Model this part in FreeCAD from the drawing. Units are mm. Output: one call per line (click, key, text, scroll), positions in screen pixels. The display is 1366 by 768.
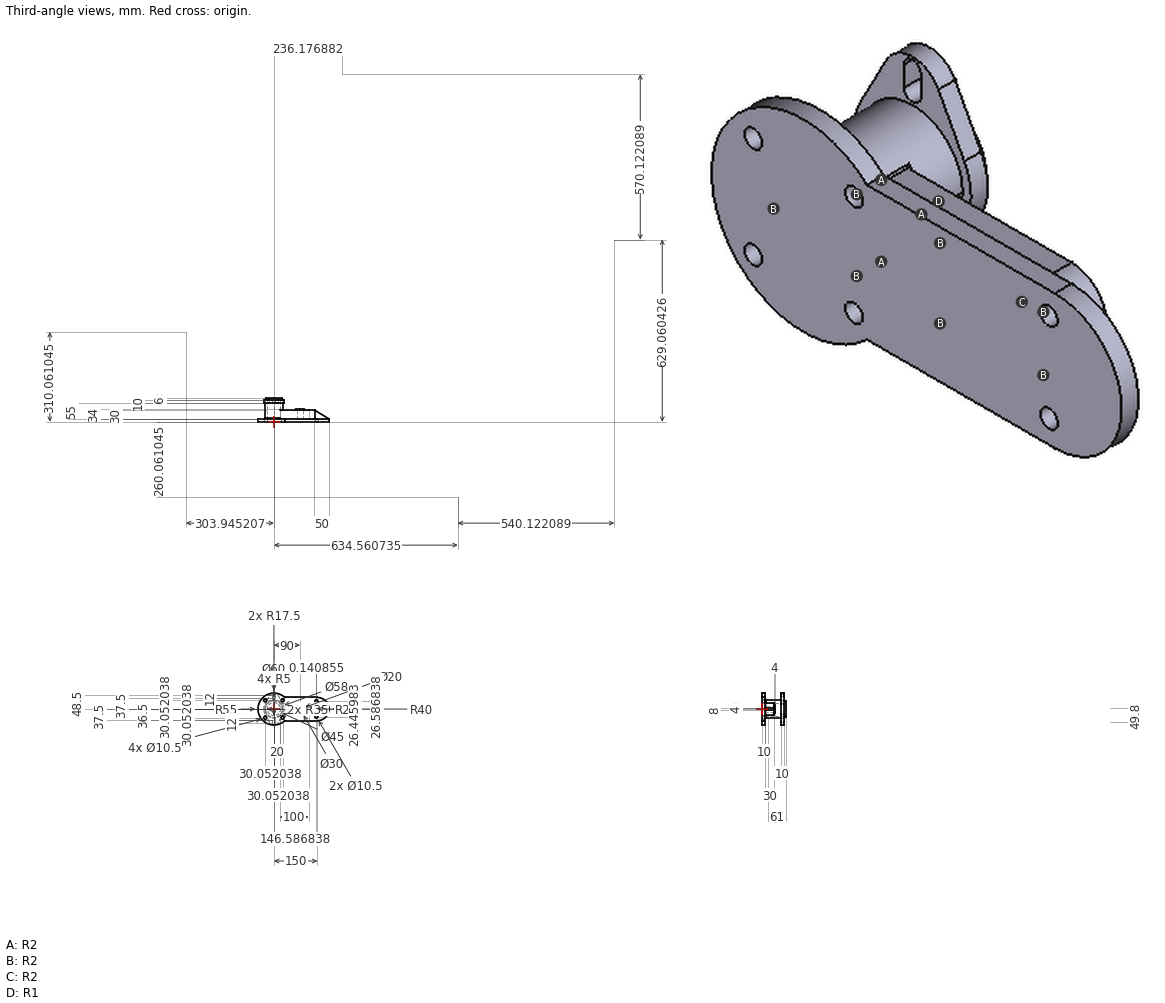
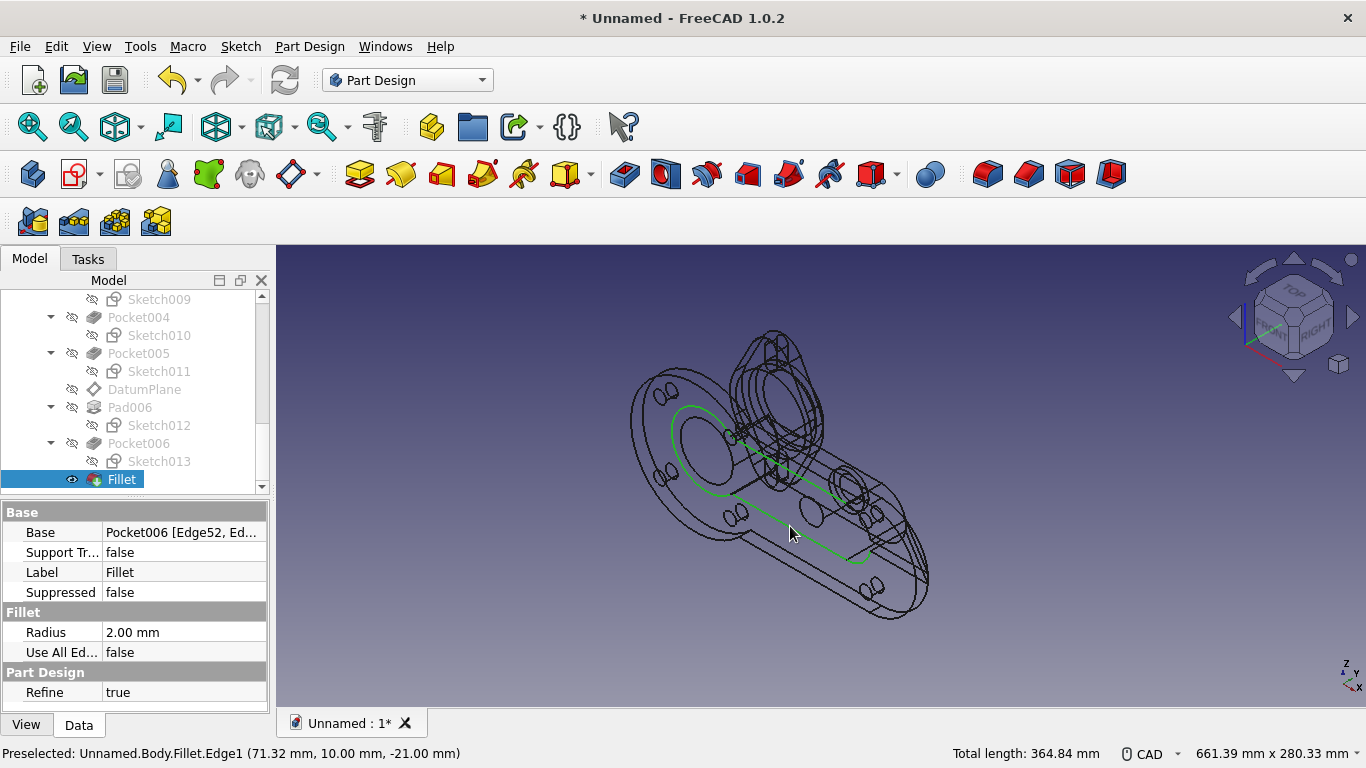
click(853, 507, ctrl)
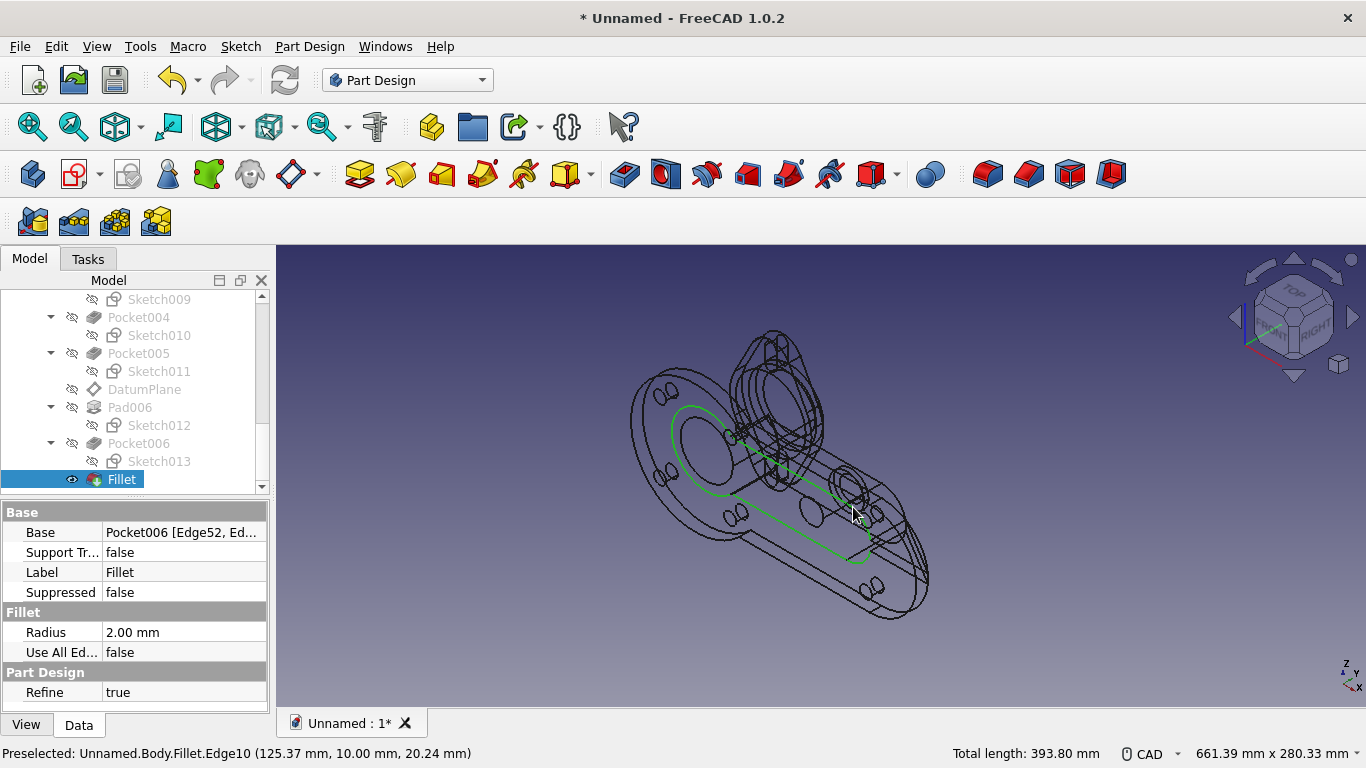
scroll(732, 493, up, 14)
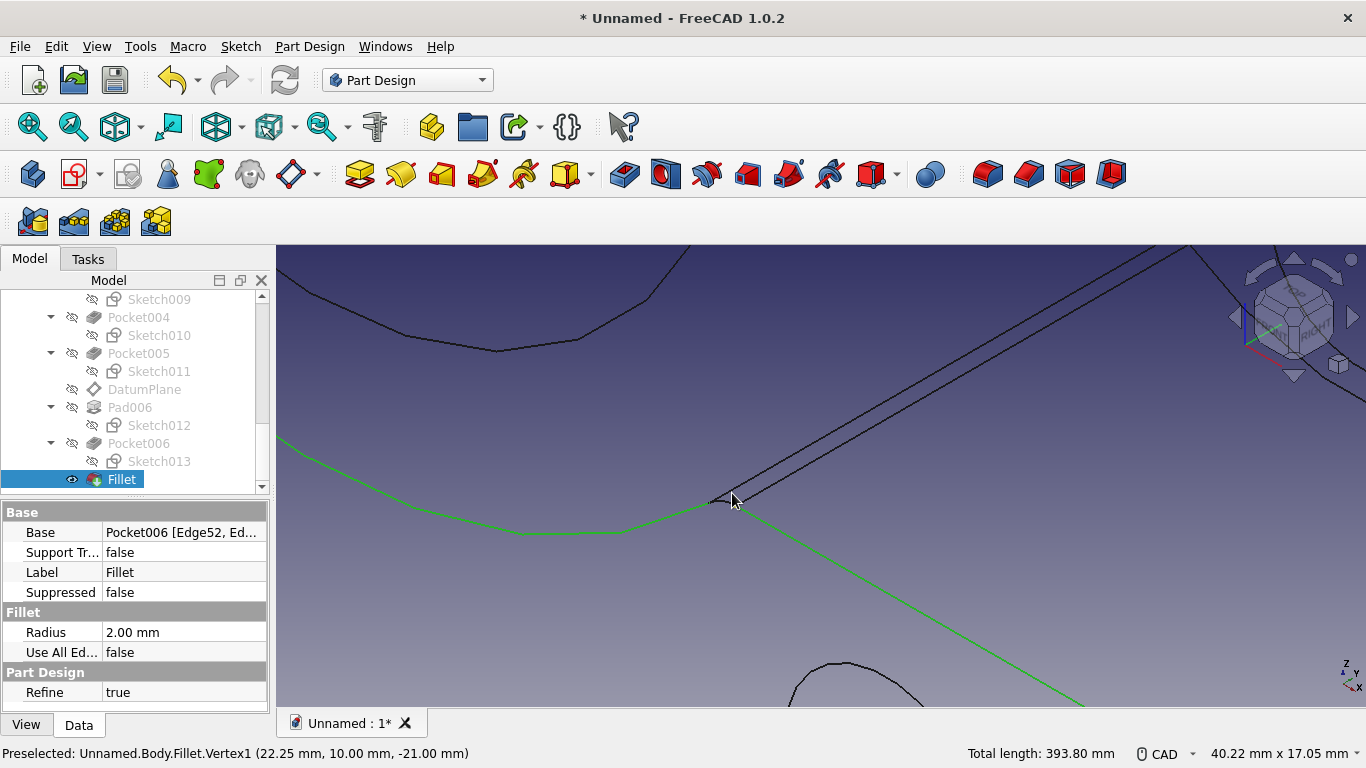
click(722, 500, ctrl)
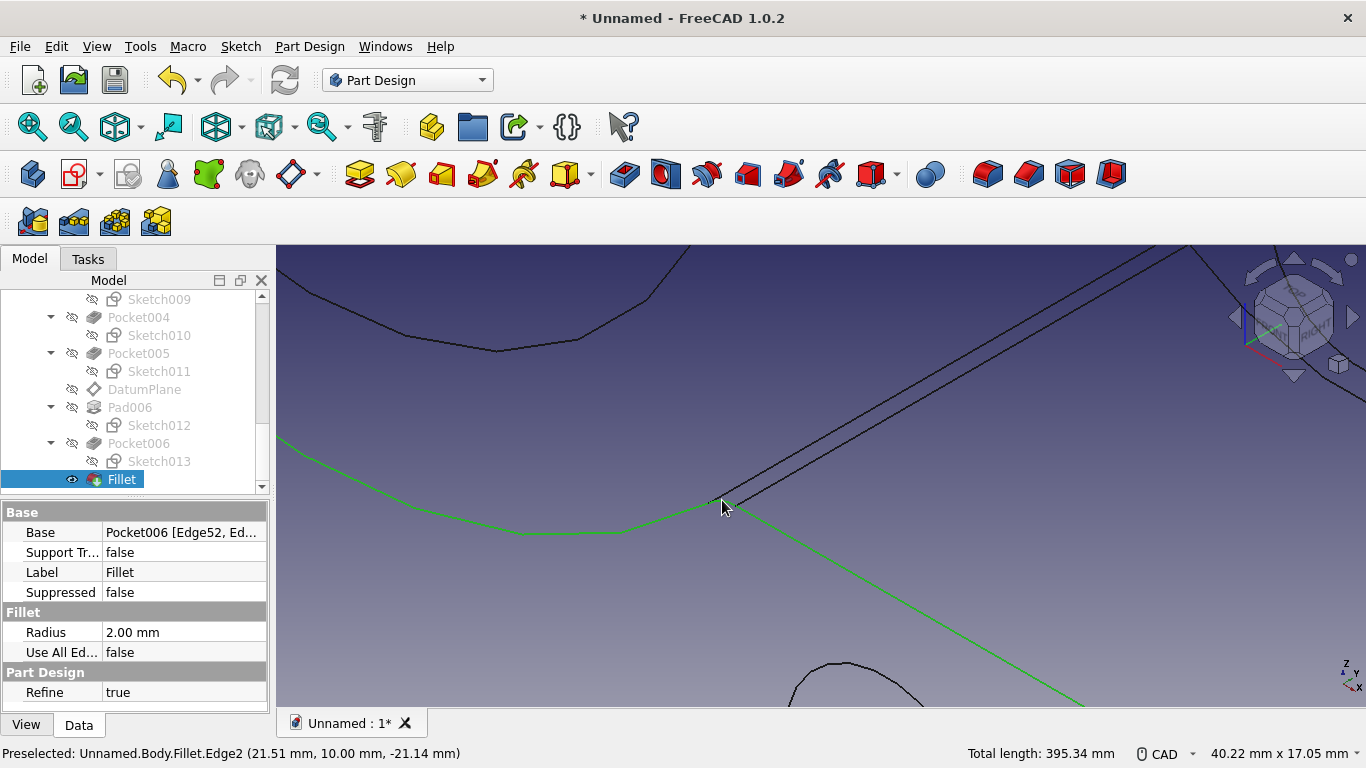
key(v)
key(f)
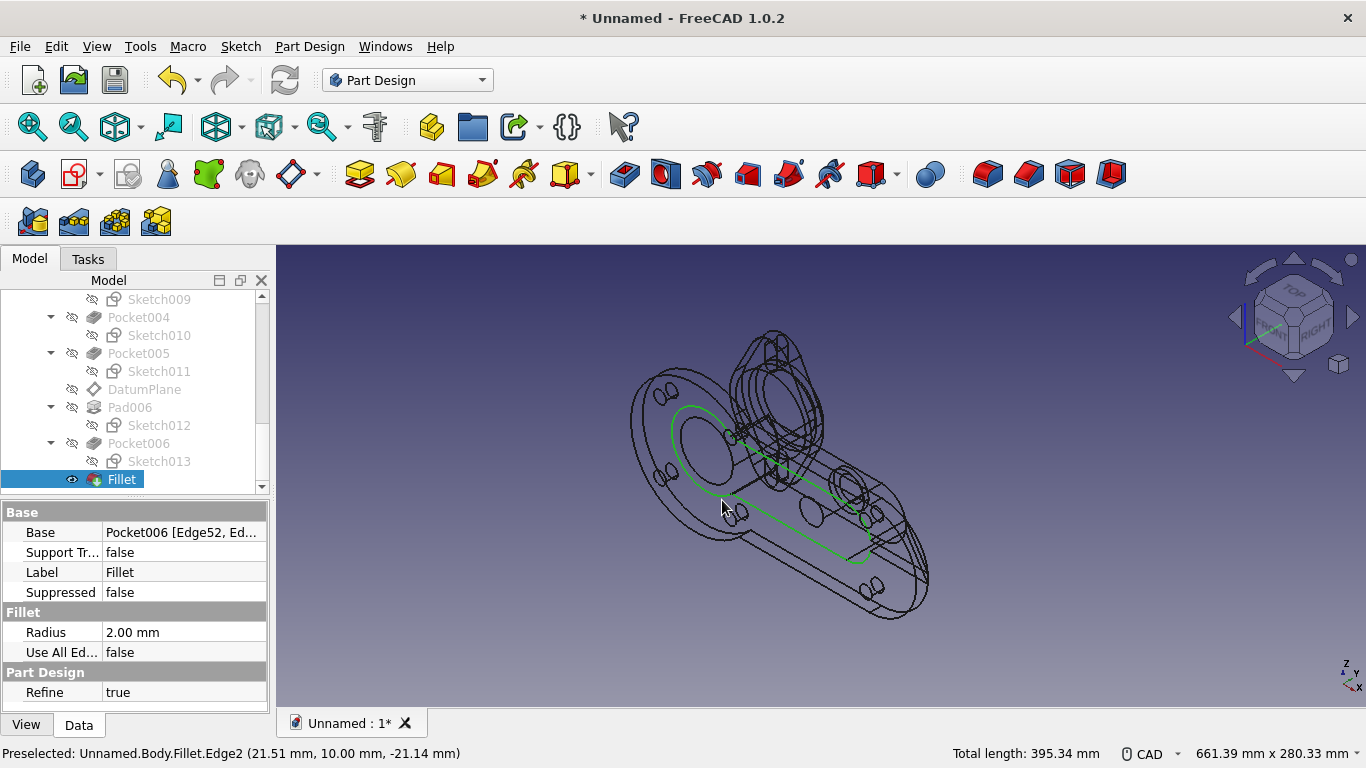
key(2)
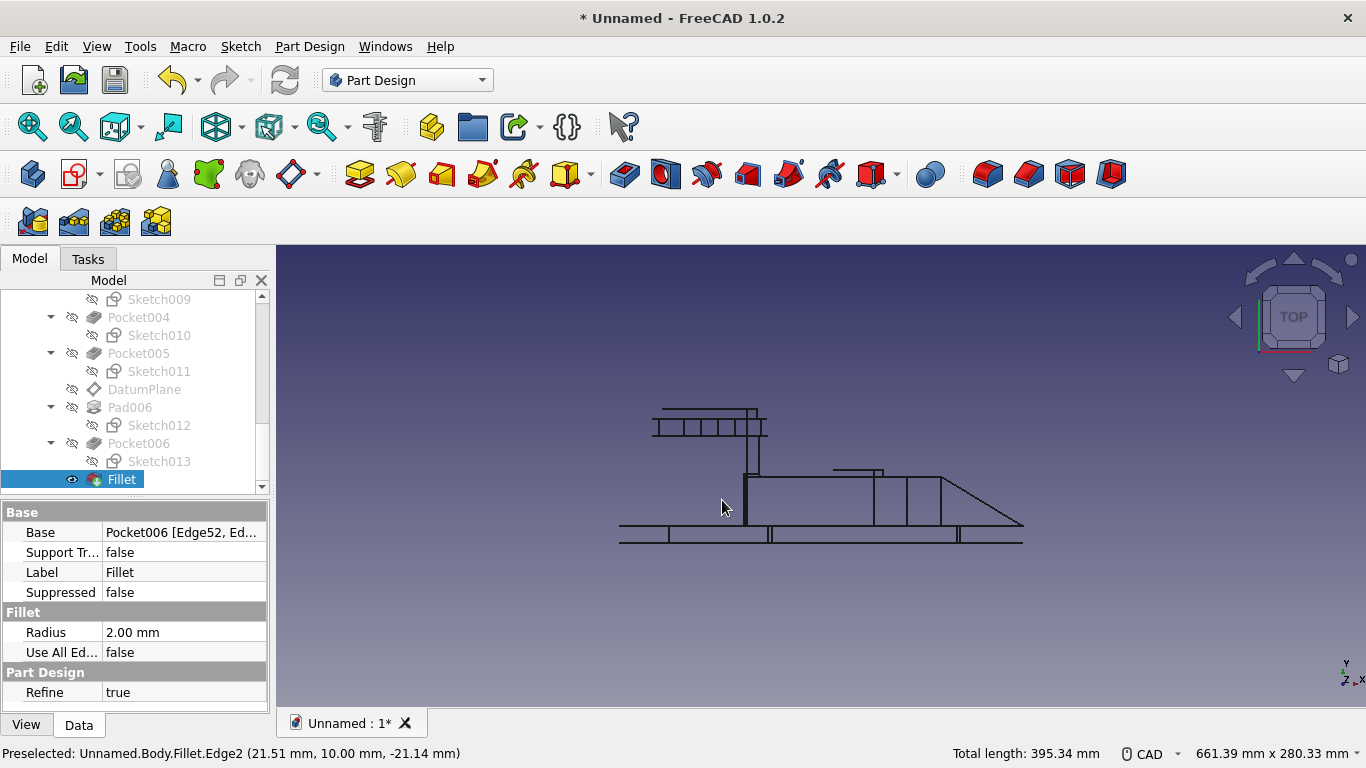
key(v)
key(f)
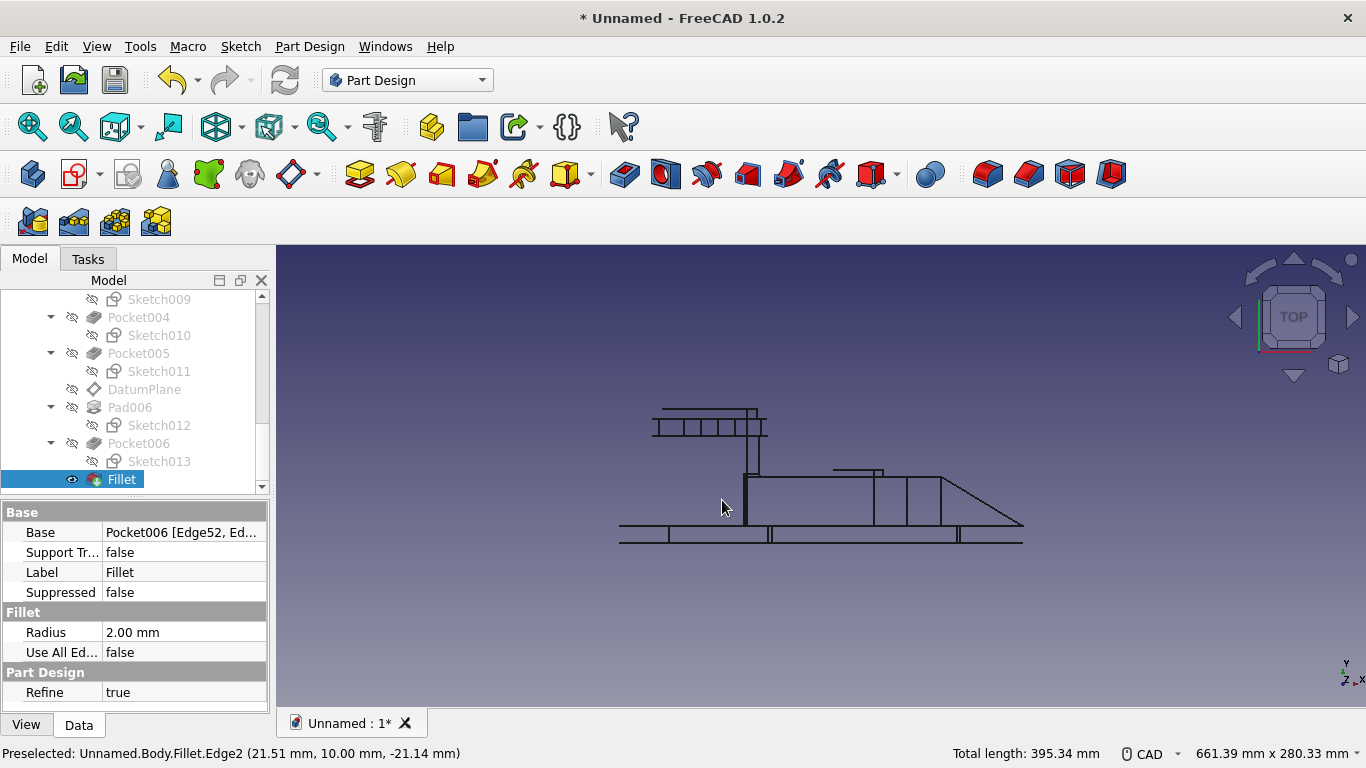
scroll(745, 525, up, 14)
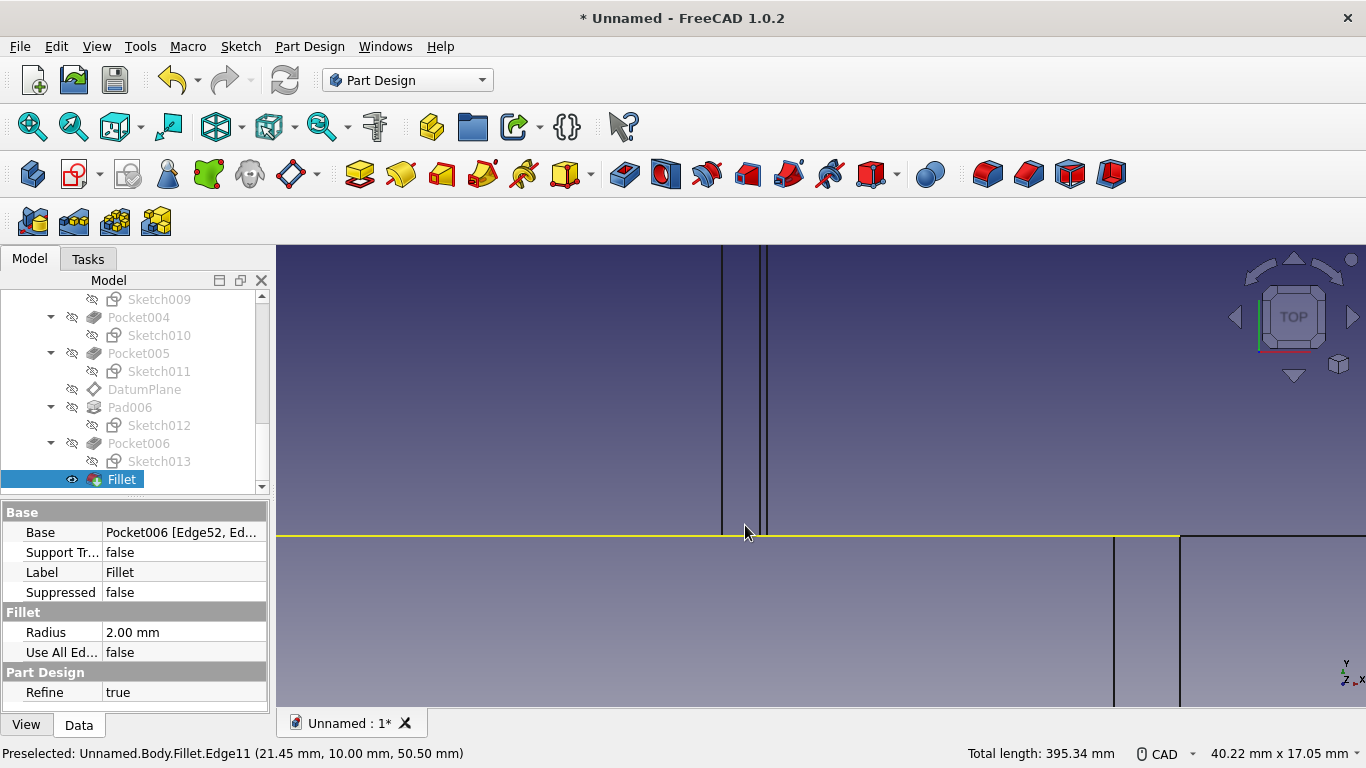
key(v)
key(f)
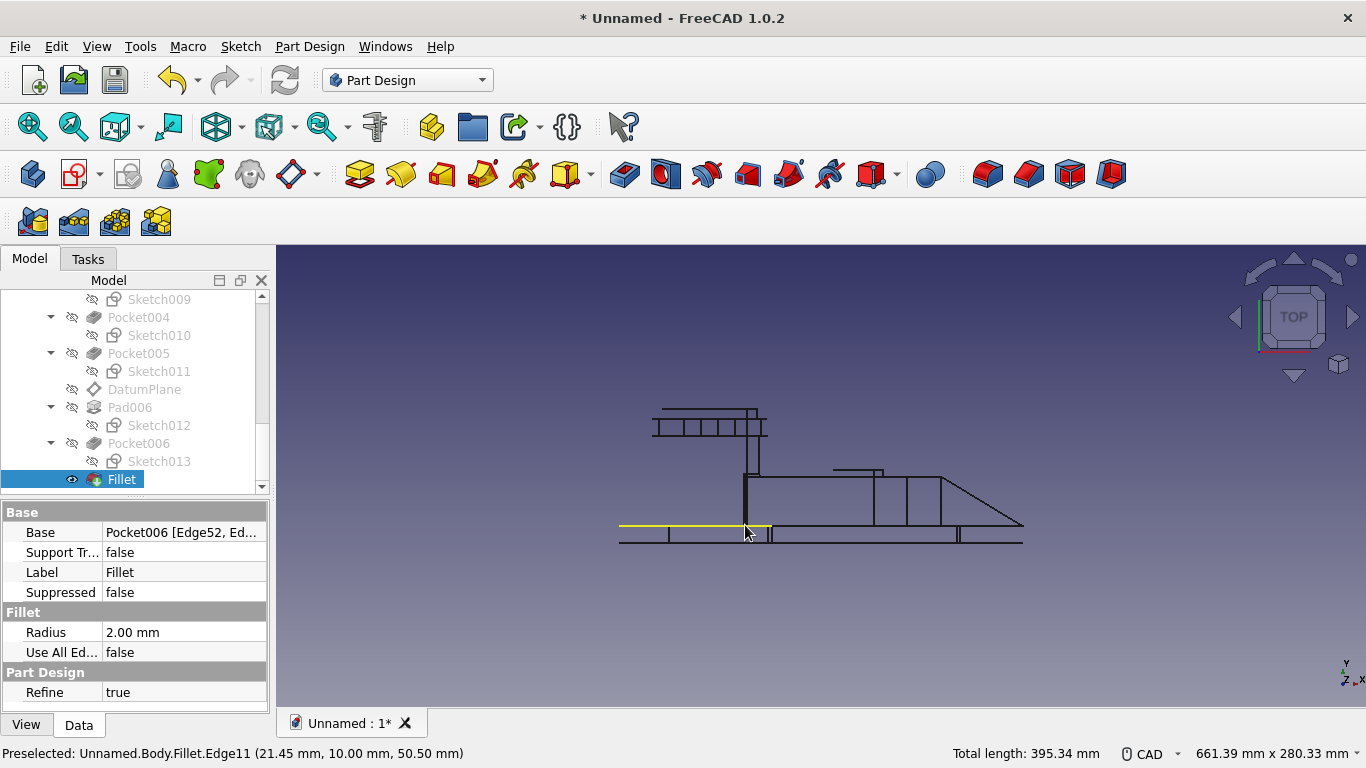
key(1)